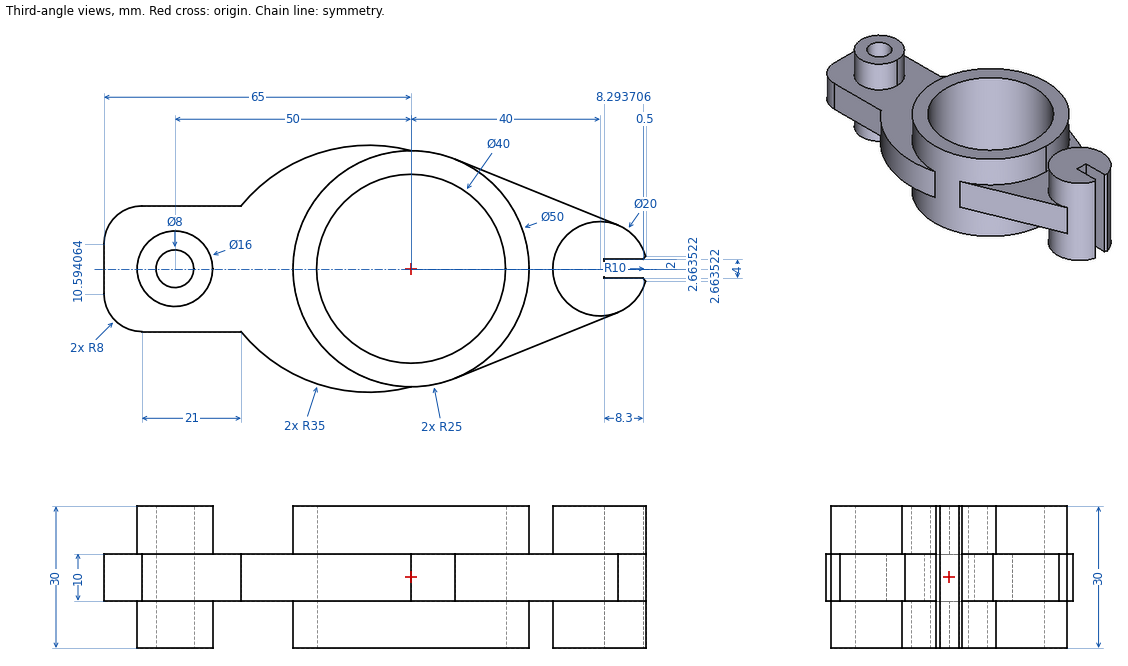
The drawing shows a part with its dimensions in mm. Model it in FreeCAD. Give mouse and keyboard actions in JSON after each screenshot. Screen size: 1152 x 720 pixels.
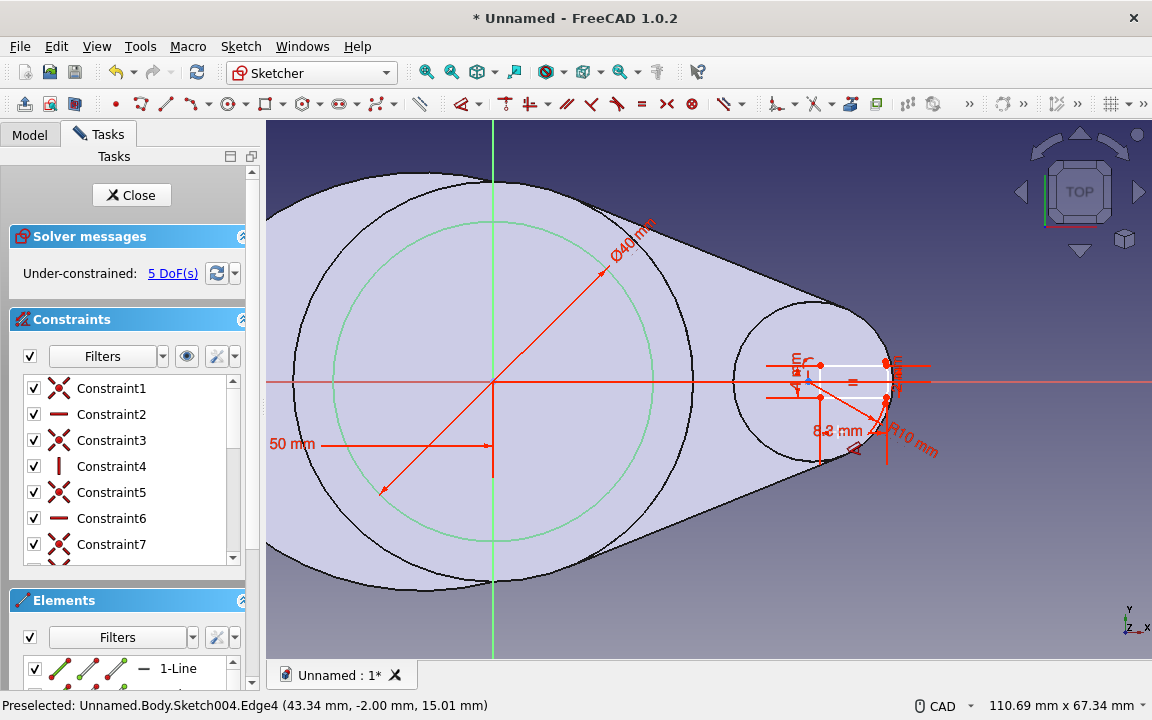
{"action": "left_click", "coordinate": [808, 382]}
{"action": "left_click", "coordinate": [578, 416]}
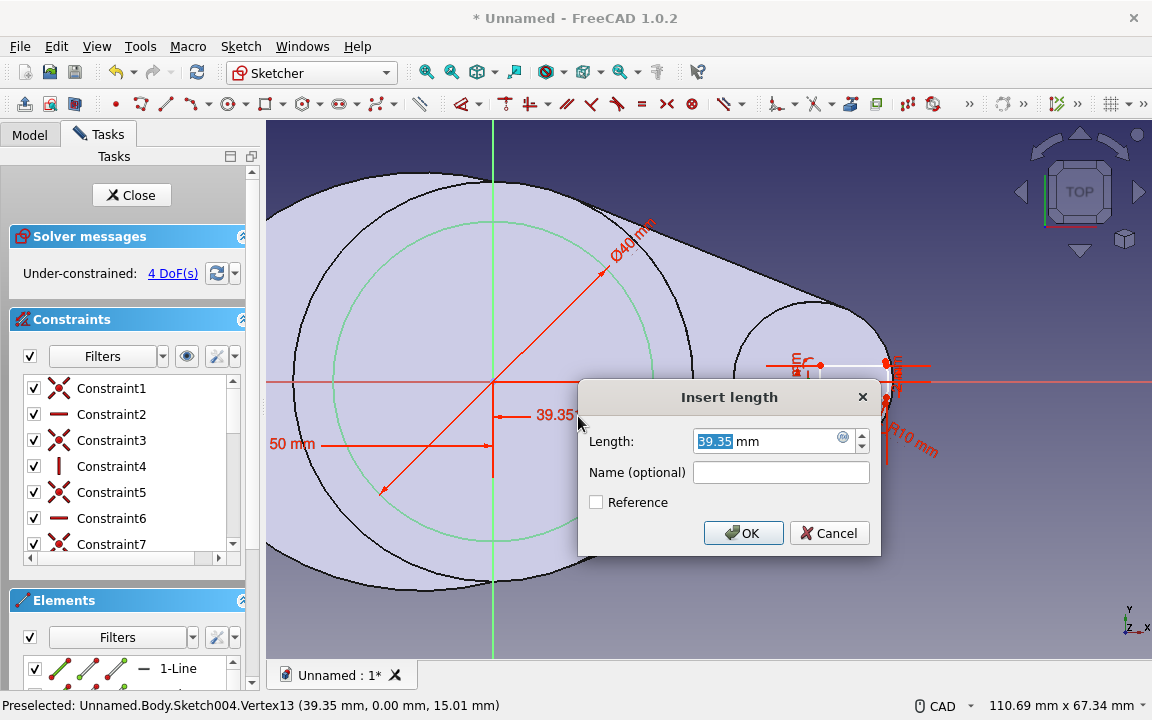
{"action": "type", "text": "40"}
{"action": "key", "text": "Return"}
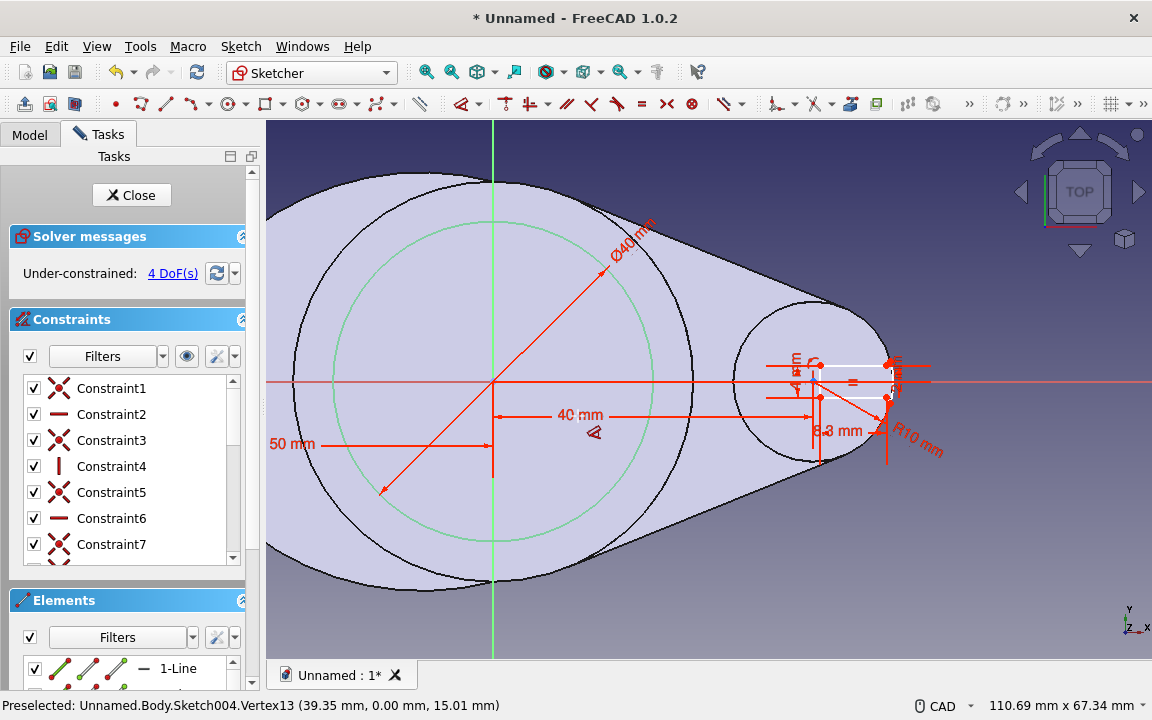
{"action": "scroll", "coordinate": [889, 364], "scroll_direction": "up", "scroll_amount": 12}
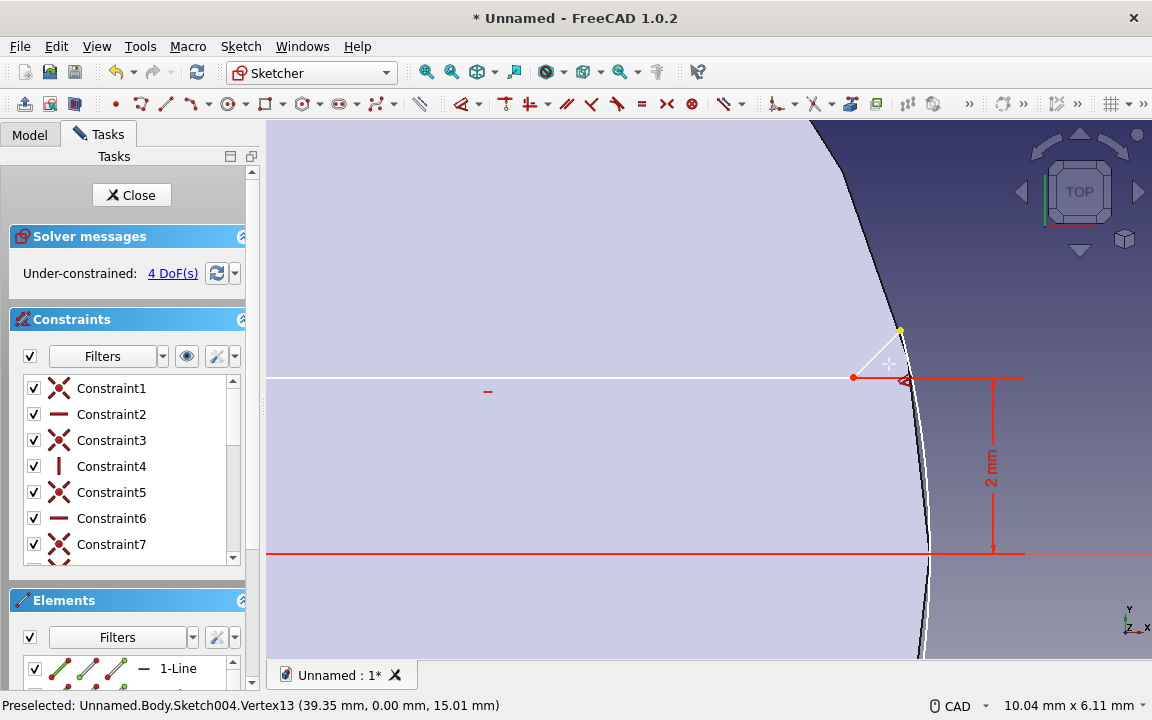
{"action": "left_click", "coordinate": [877, 354]}
{"action": "left_click", "coordinate": [877, 296]}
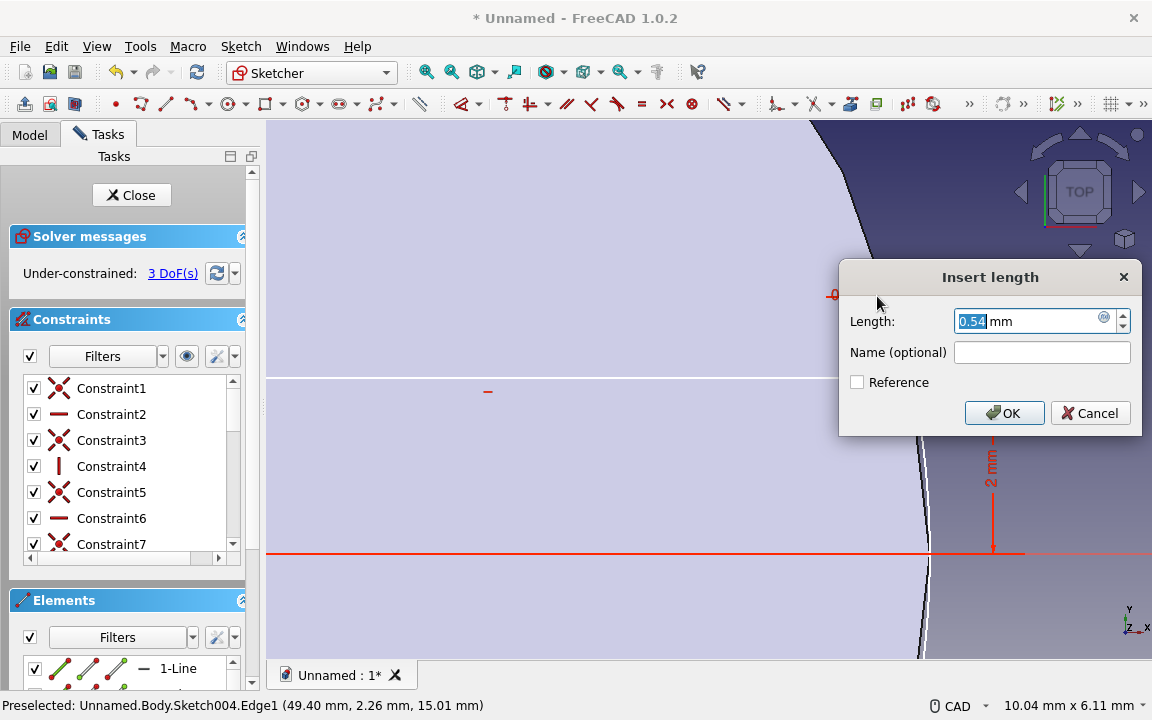
{"action": "type", "text": "0.5"}
{"action": "key", "text": "Return"}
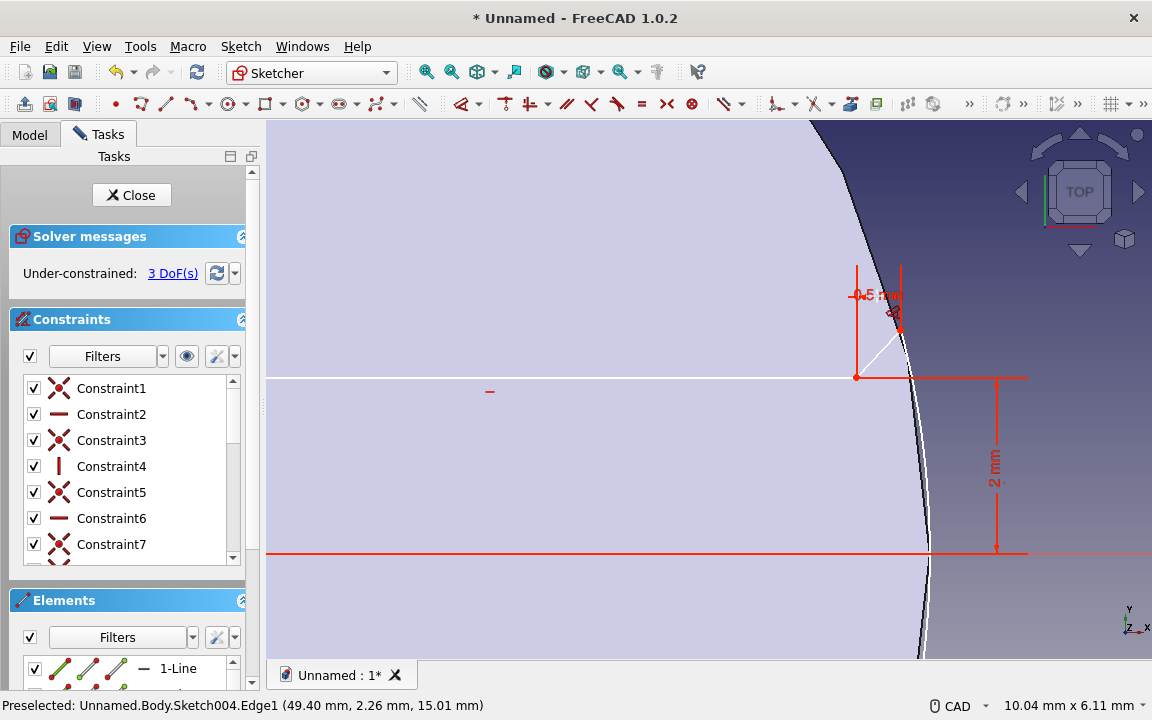
{"action": "scroll", "coordinate": [866, 381], "scroll_direction": "down", "scroll_amount": 15}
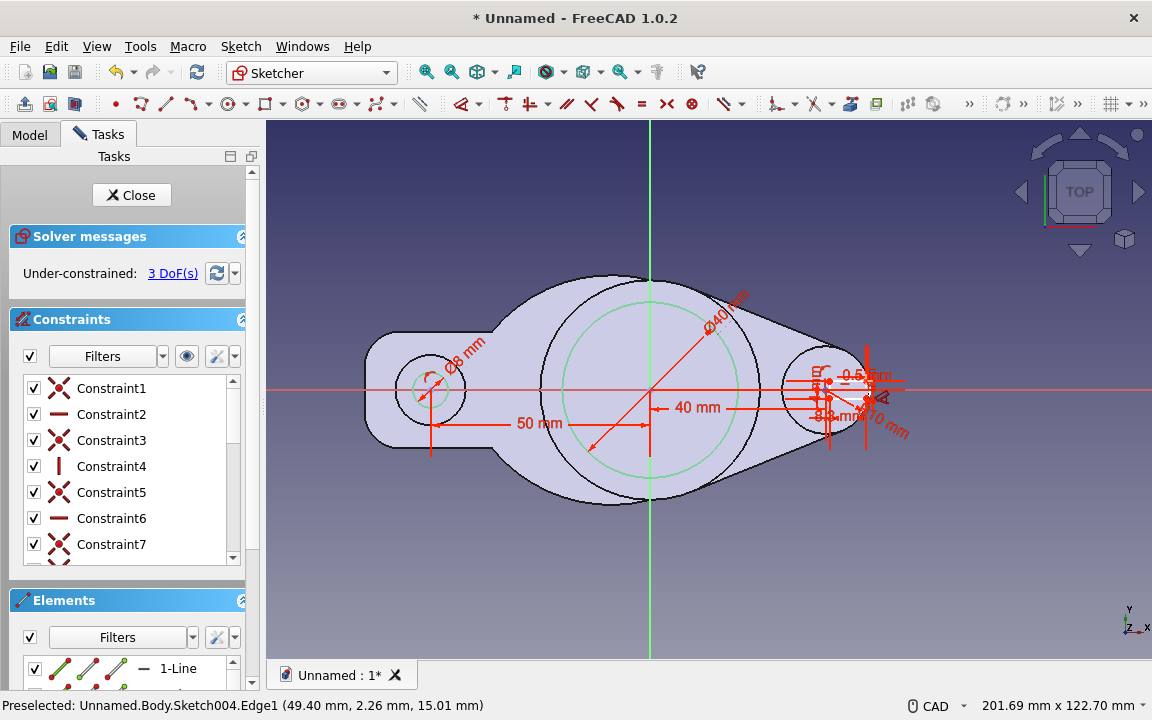
{"action": "scroll", "coordinate": [855, 381], "scroll_direction": "up", "scroll_amount": 3}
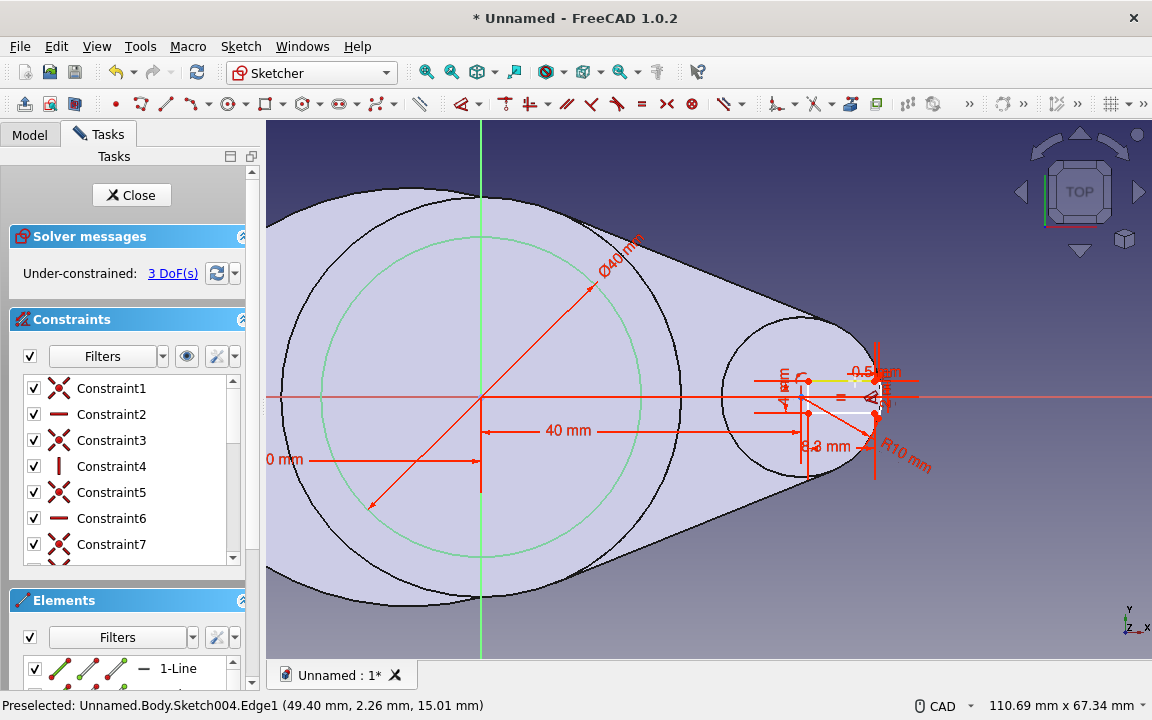
{"action": "left_click", "coordinate": [855, 381]}
{"action": "left_click", "coordinate": [842, 347]}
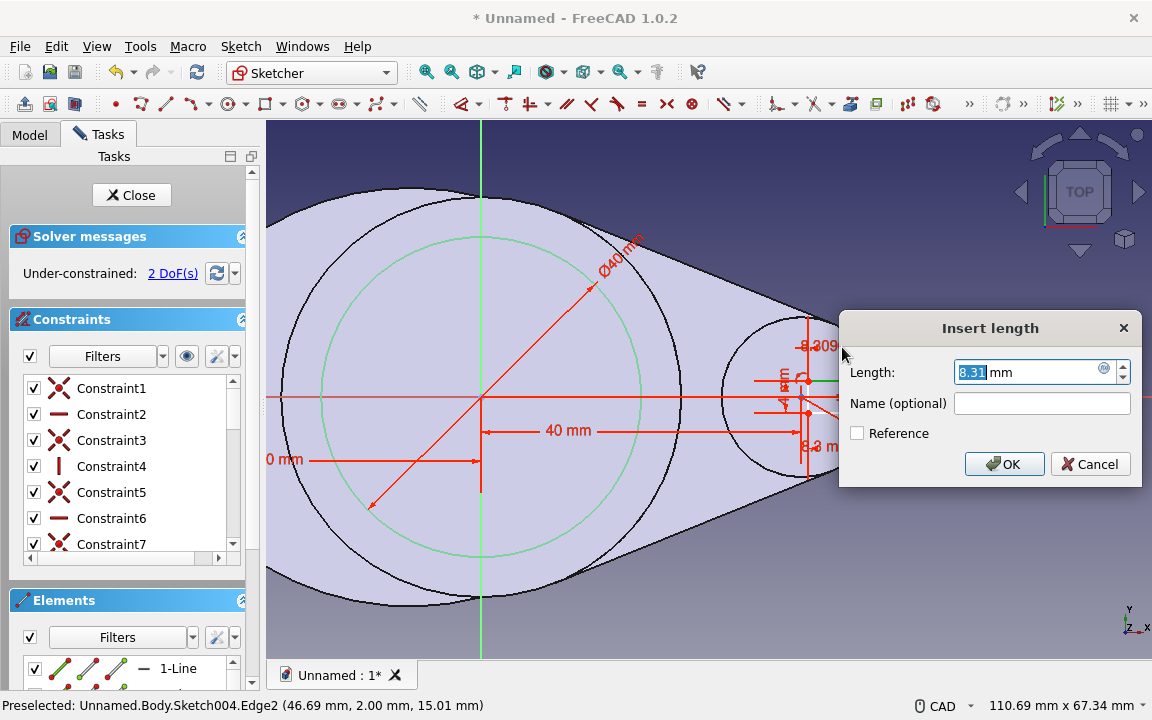
{"action": "type", "text": "8.293706"}
{"action": "key", "text": "Return"}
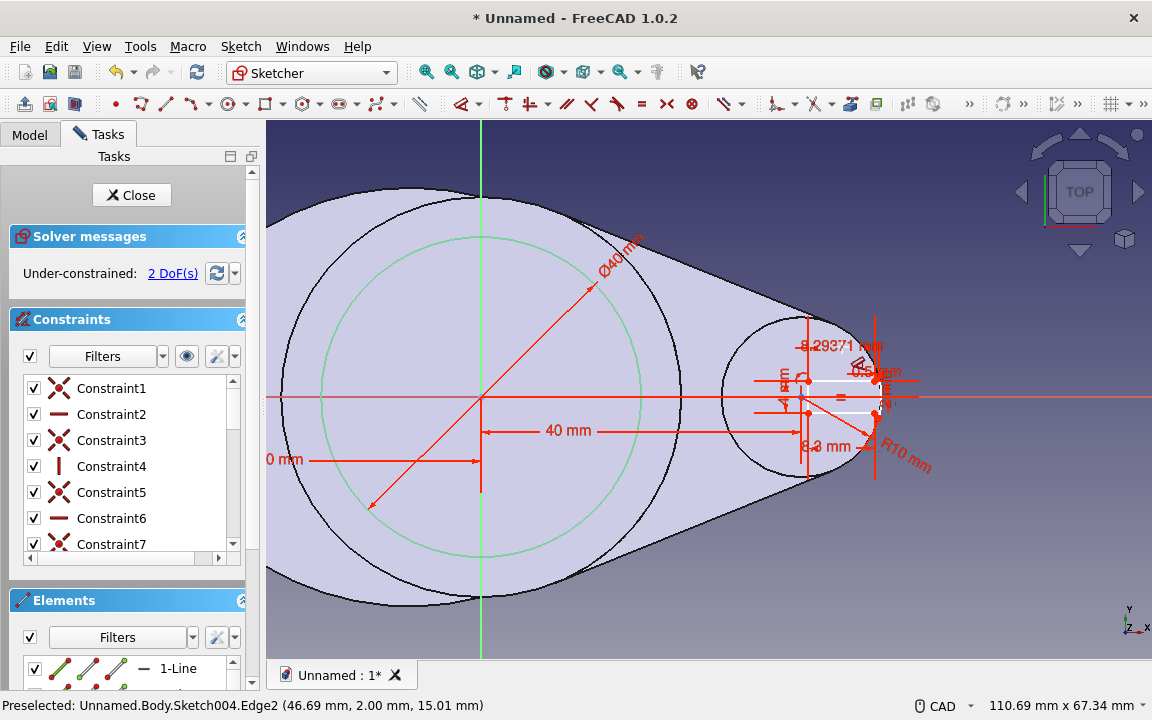
{"action": "scroll", "coordinate": [879, 377], "scroll_direction": "up", "scroll_amount": 4}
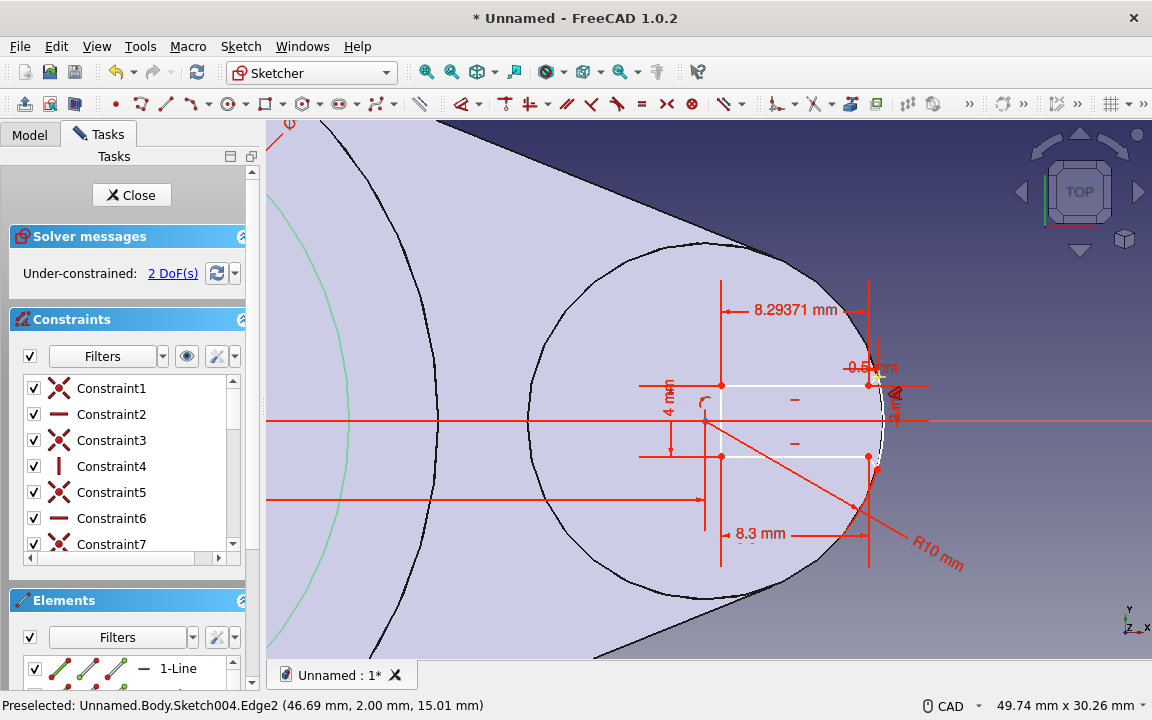
{"action": "left_click", "coordinate": [878, 376]}
{"action": "left_click", "coordinate": [960, 383]}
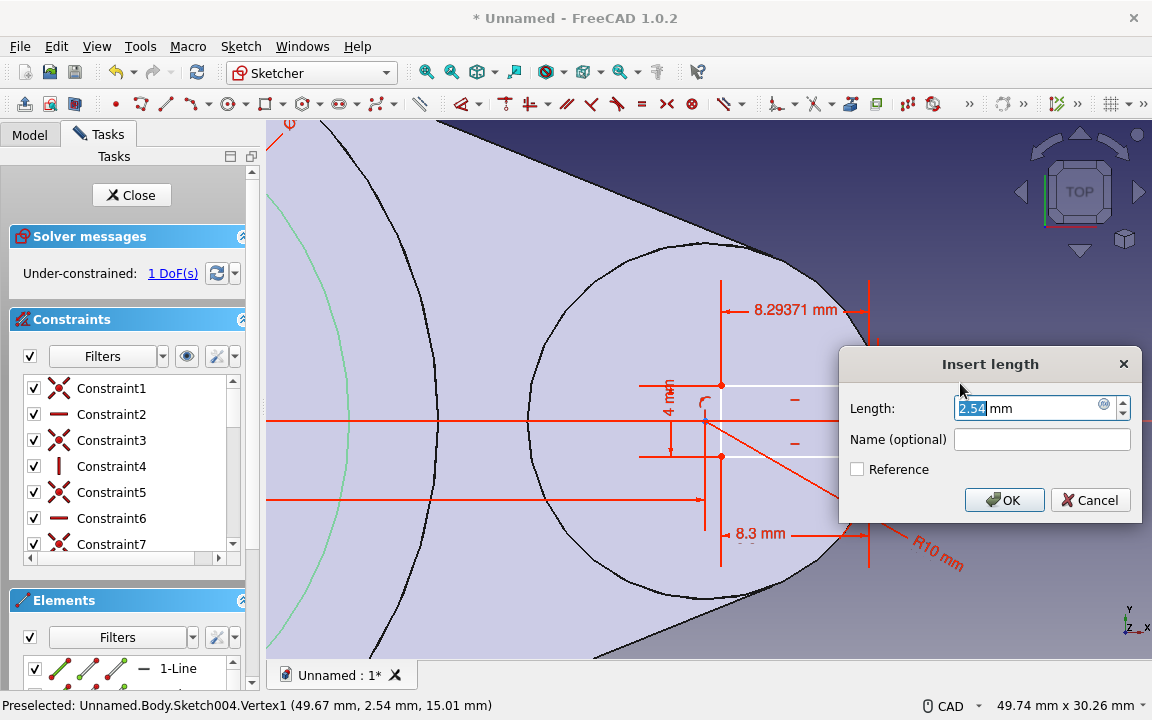
{"action": "type", "text": "2.663522"}
{"action": "key", "text": "Return"}